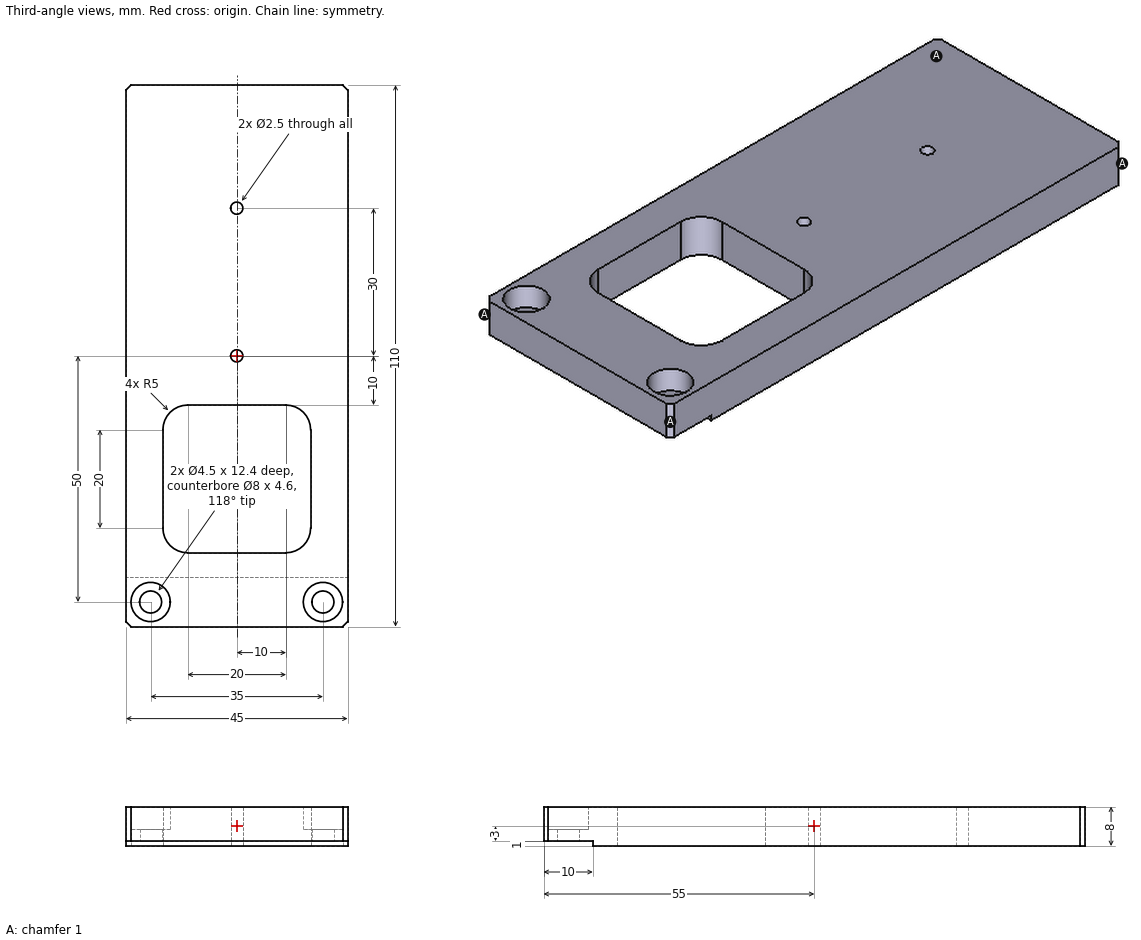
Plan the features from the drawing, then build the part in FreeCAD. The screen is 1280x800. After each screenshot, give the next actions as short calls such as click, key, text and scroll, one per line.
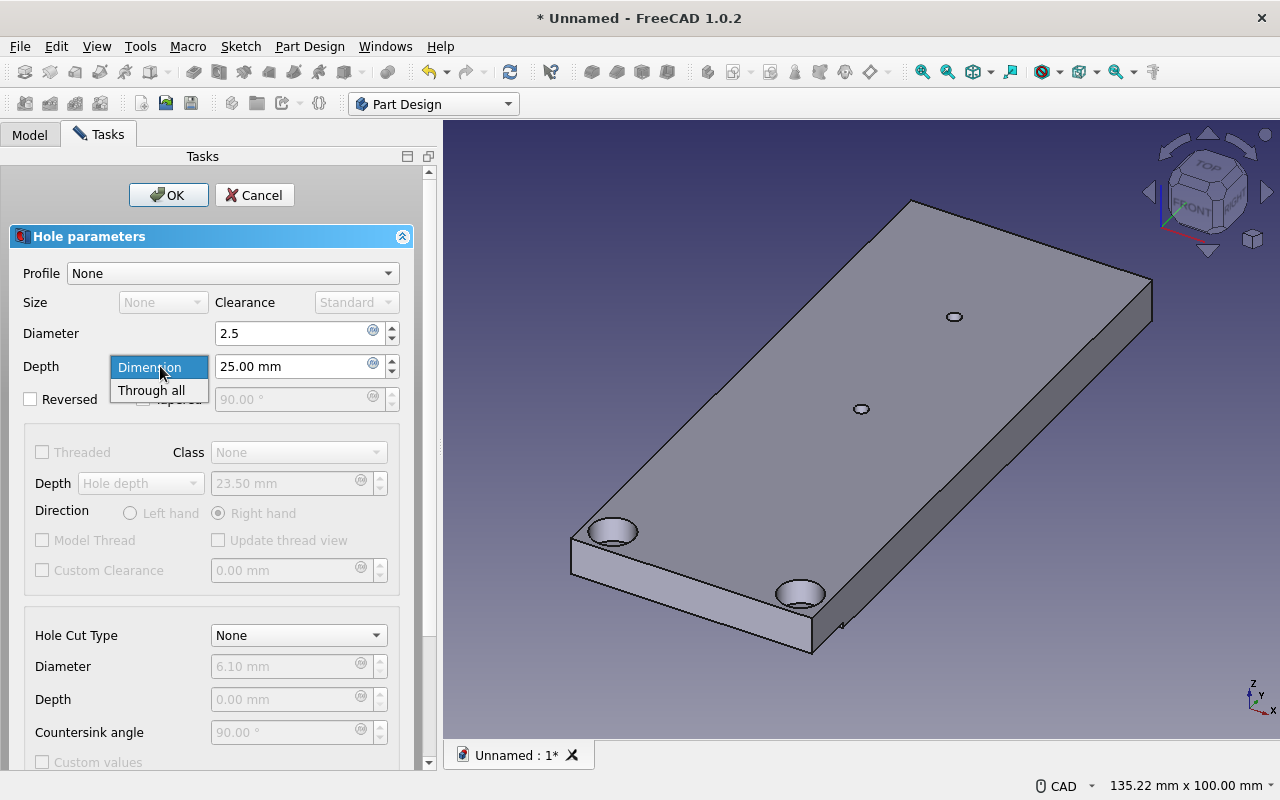
click(158, 390)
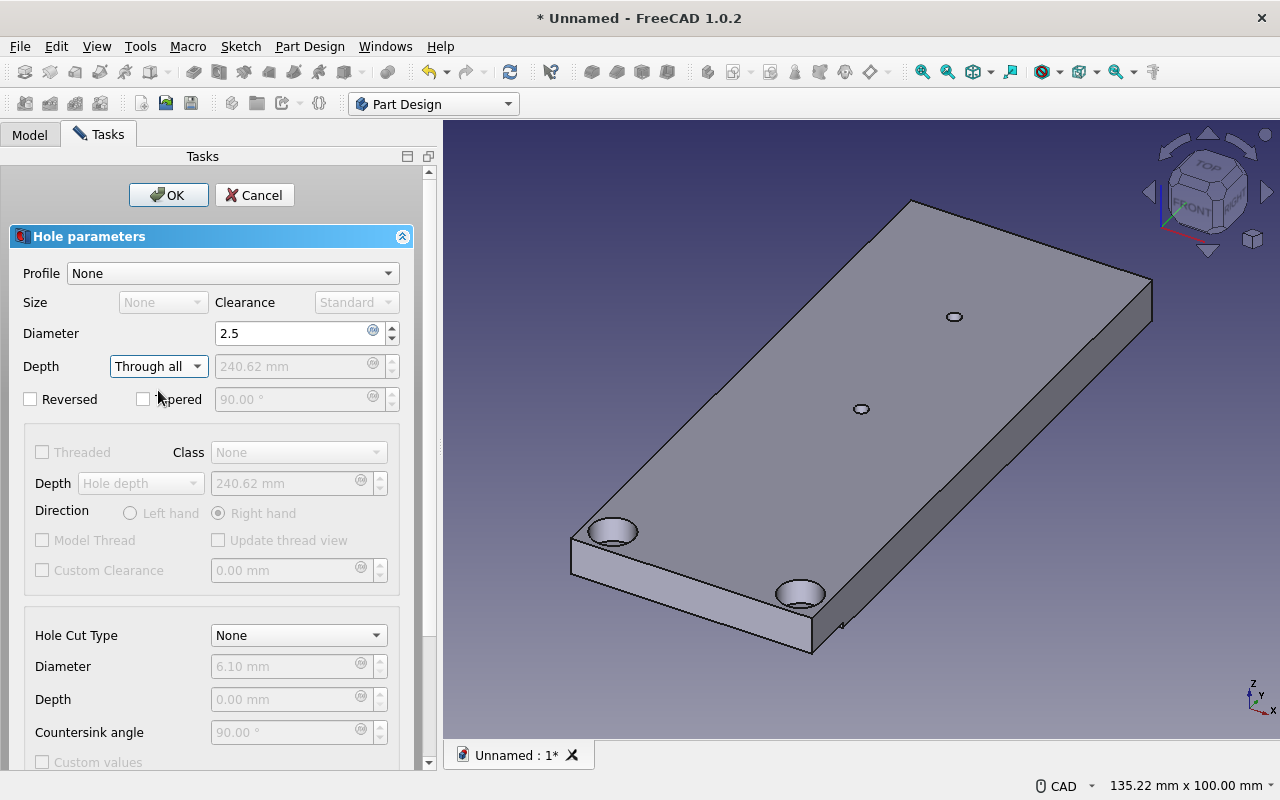
click(169, 195)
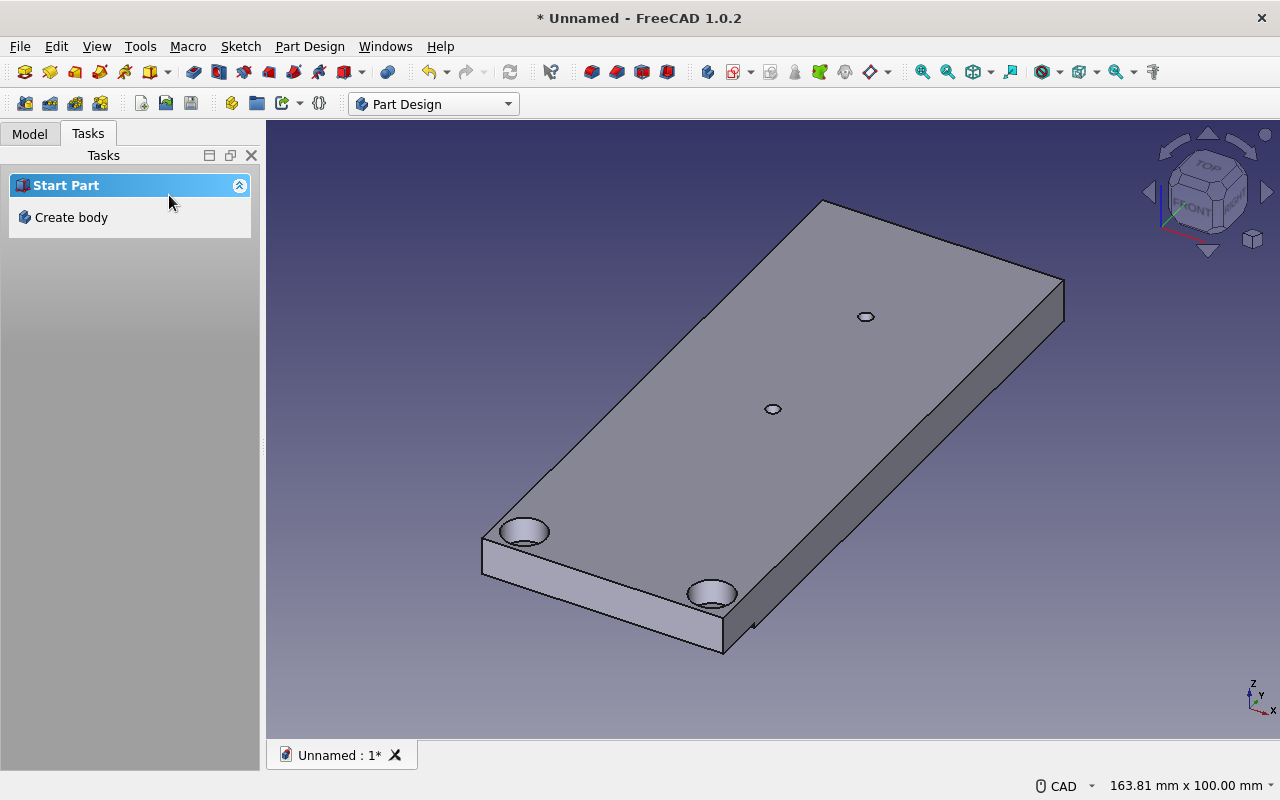
click(723, 635)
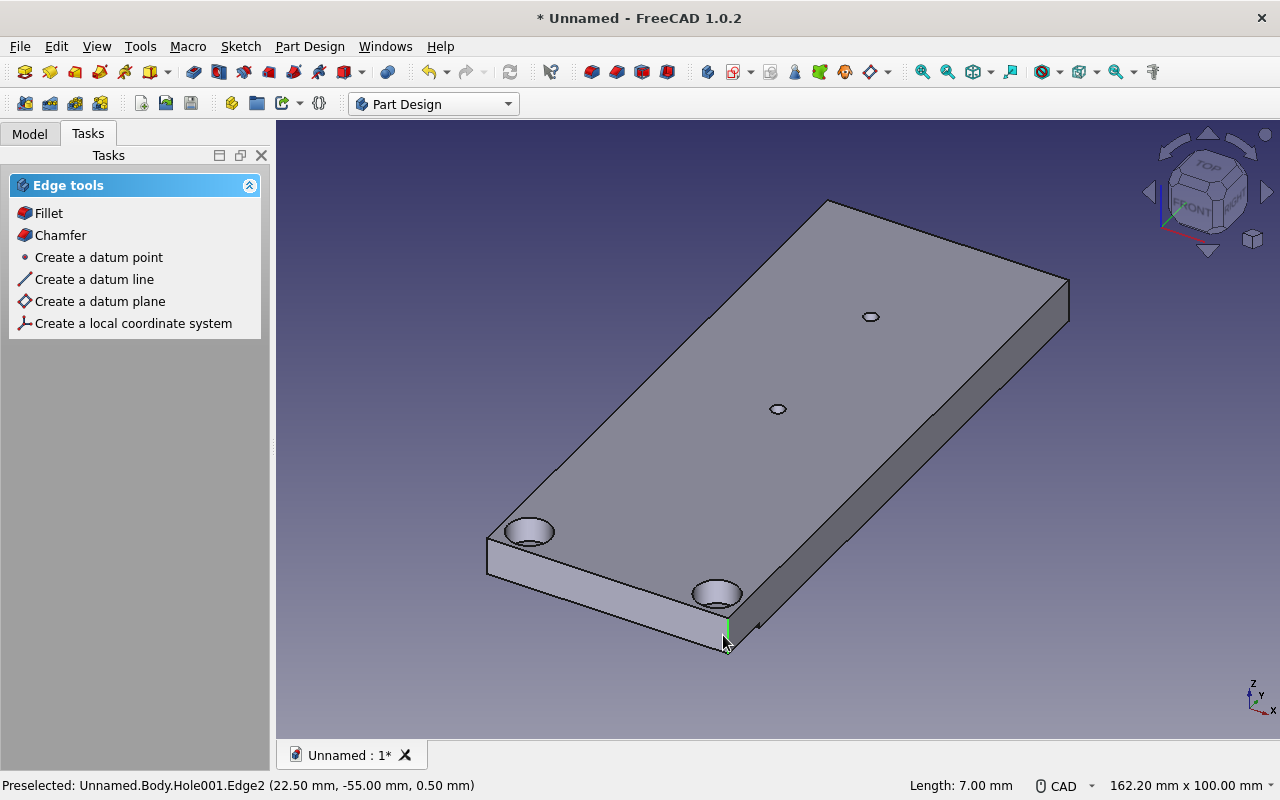
key(0)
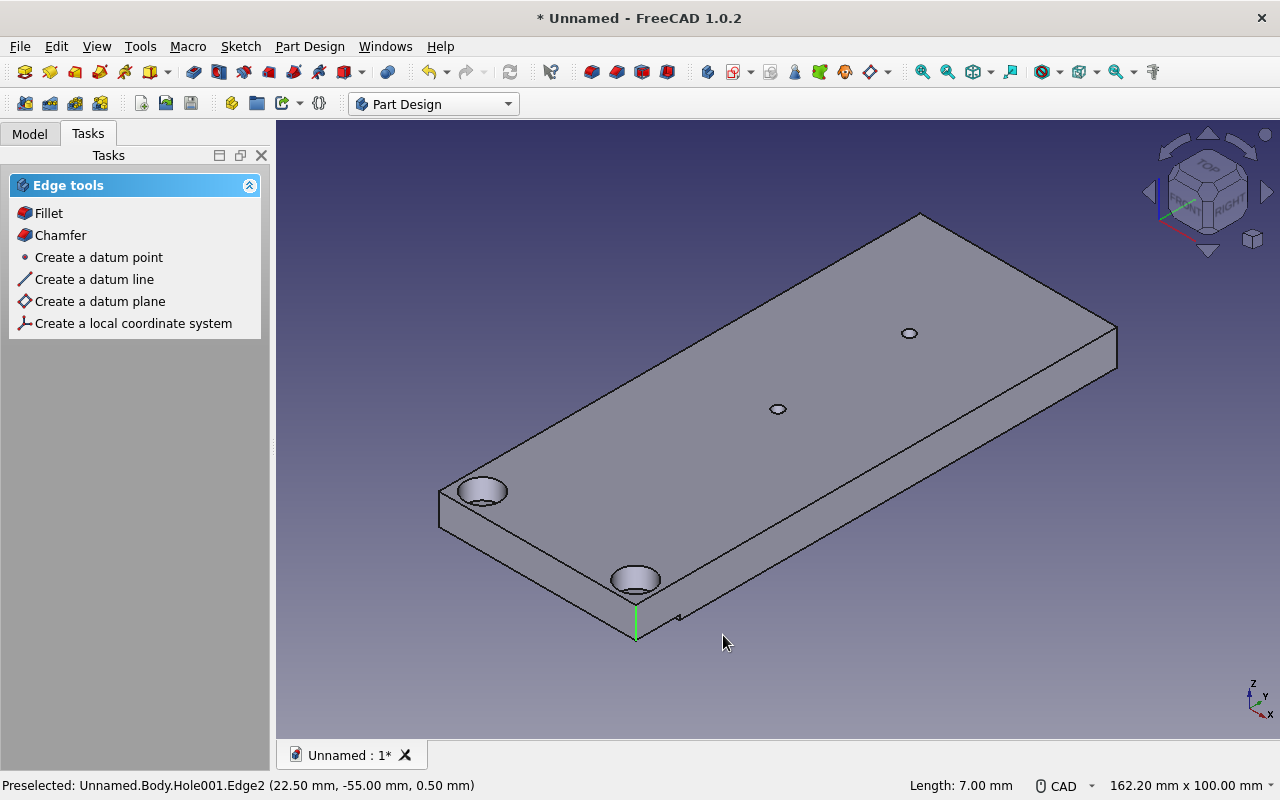
key(2)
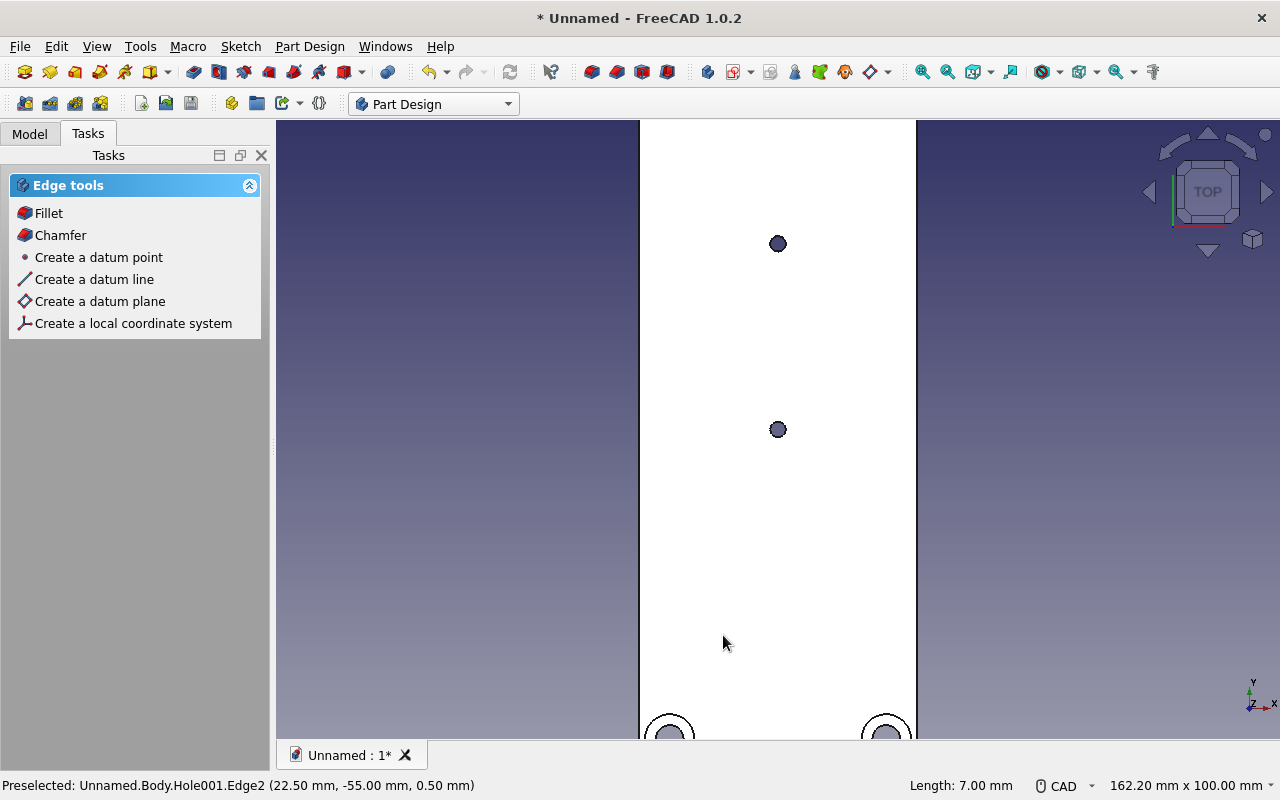
click(923, 72)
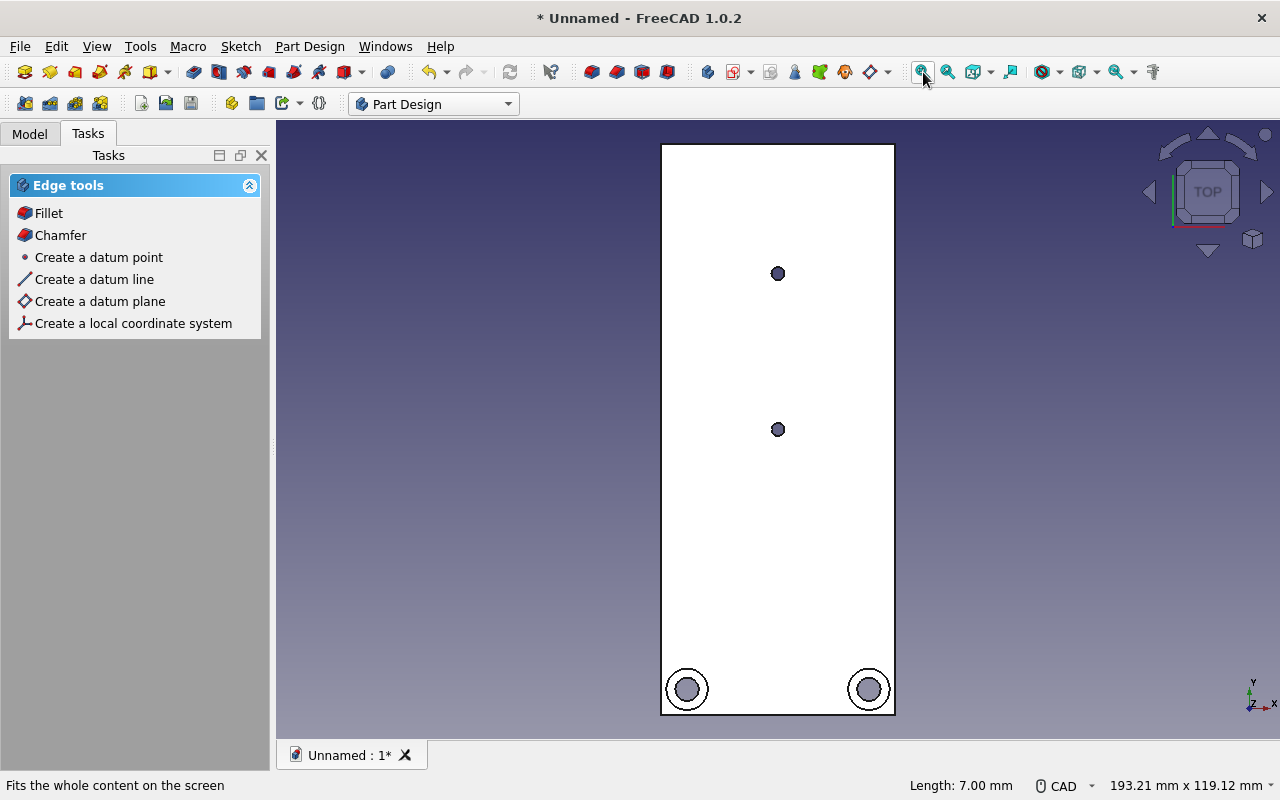
key(1)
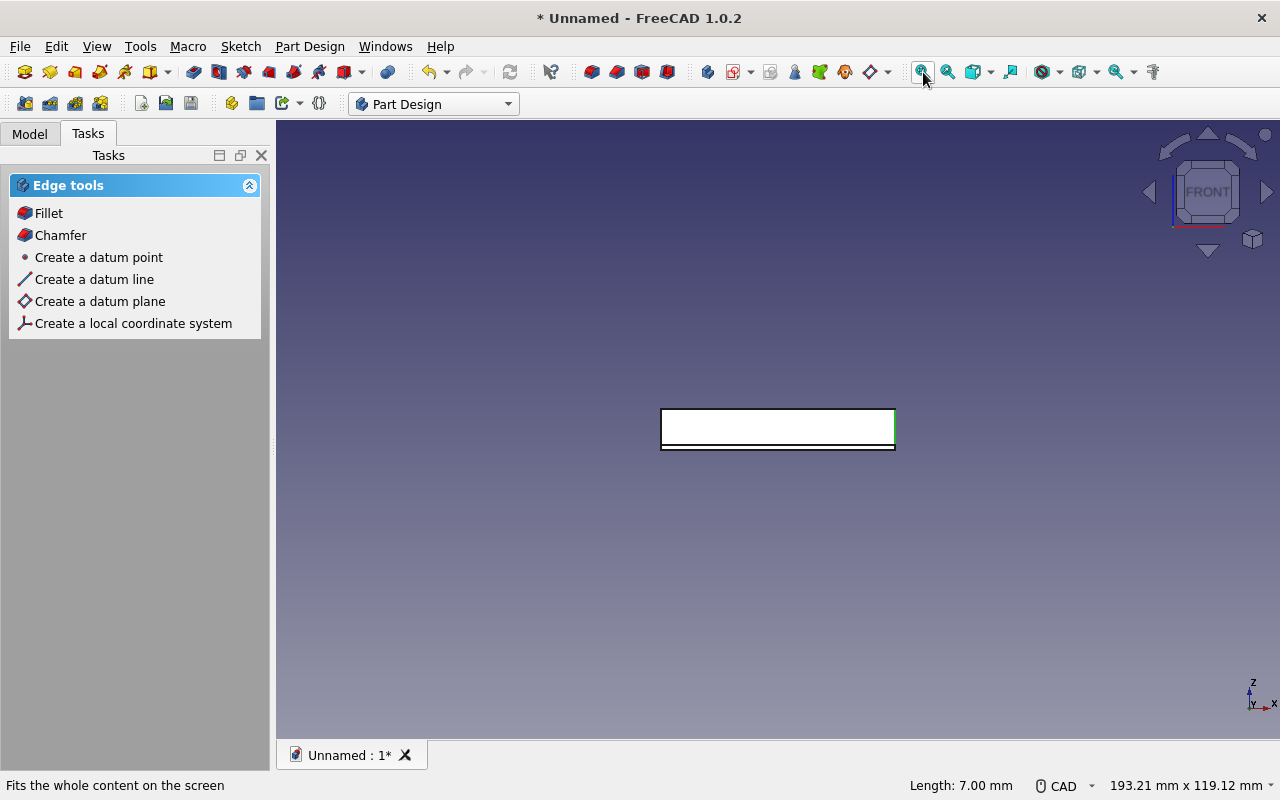
click(923, 72)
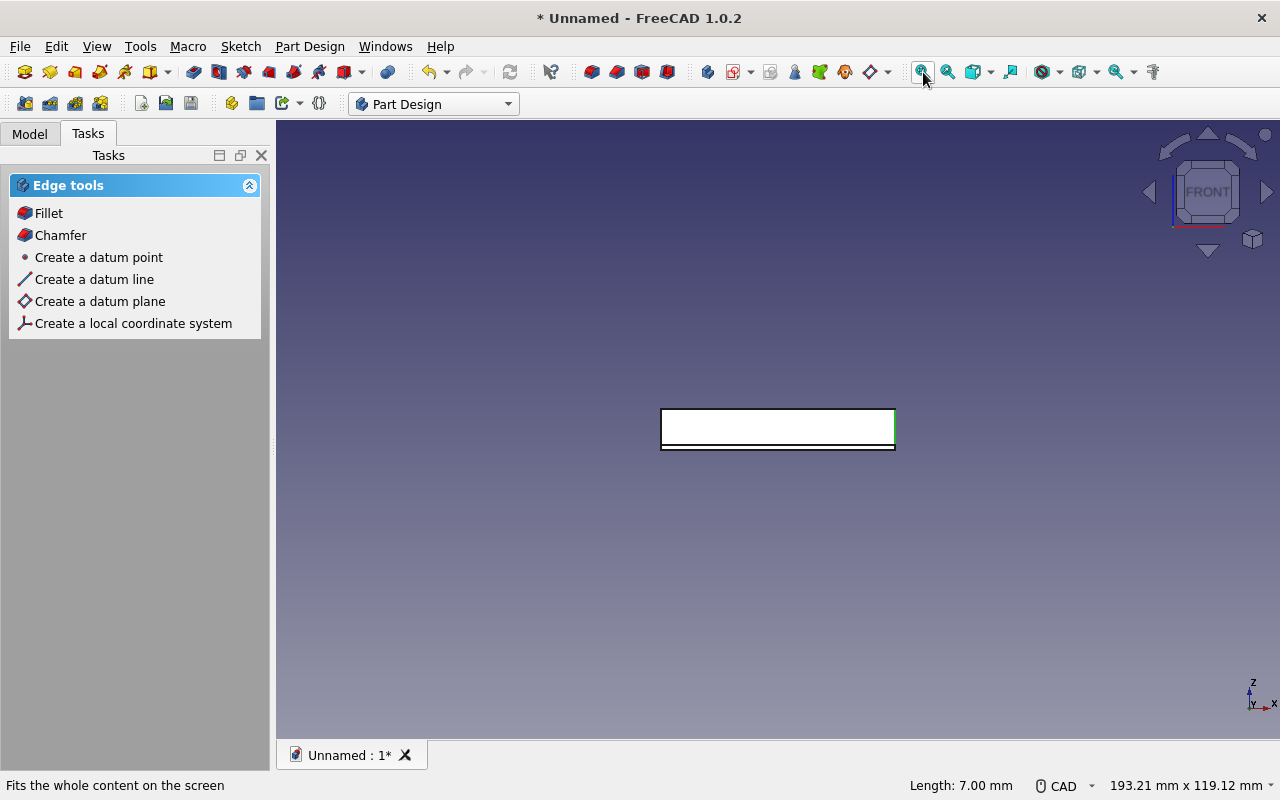
click(661, 426, ctrl)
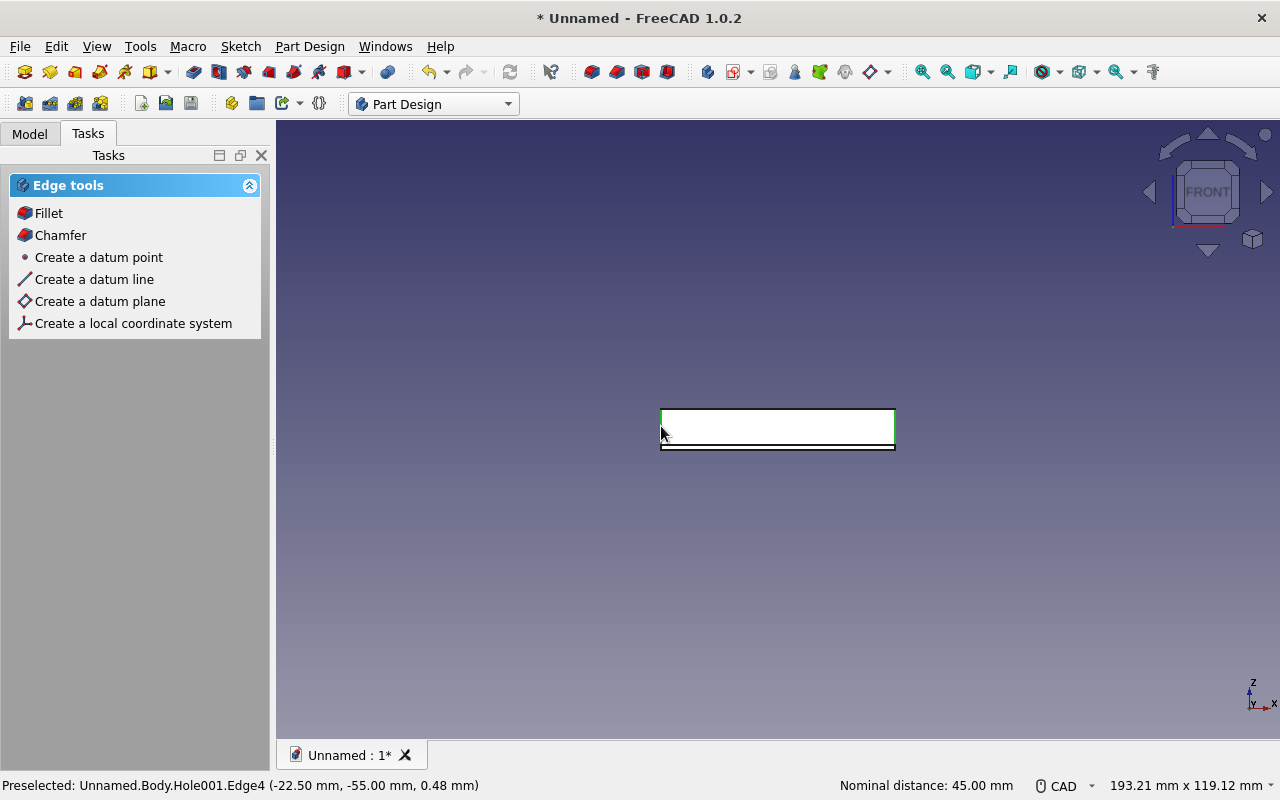
key(3)